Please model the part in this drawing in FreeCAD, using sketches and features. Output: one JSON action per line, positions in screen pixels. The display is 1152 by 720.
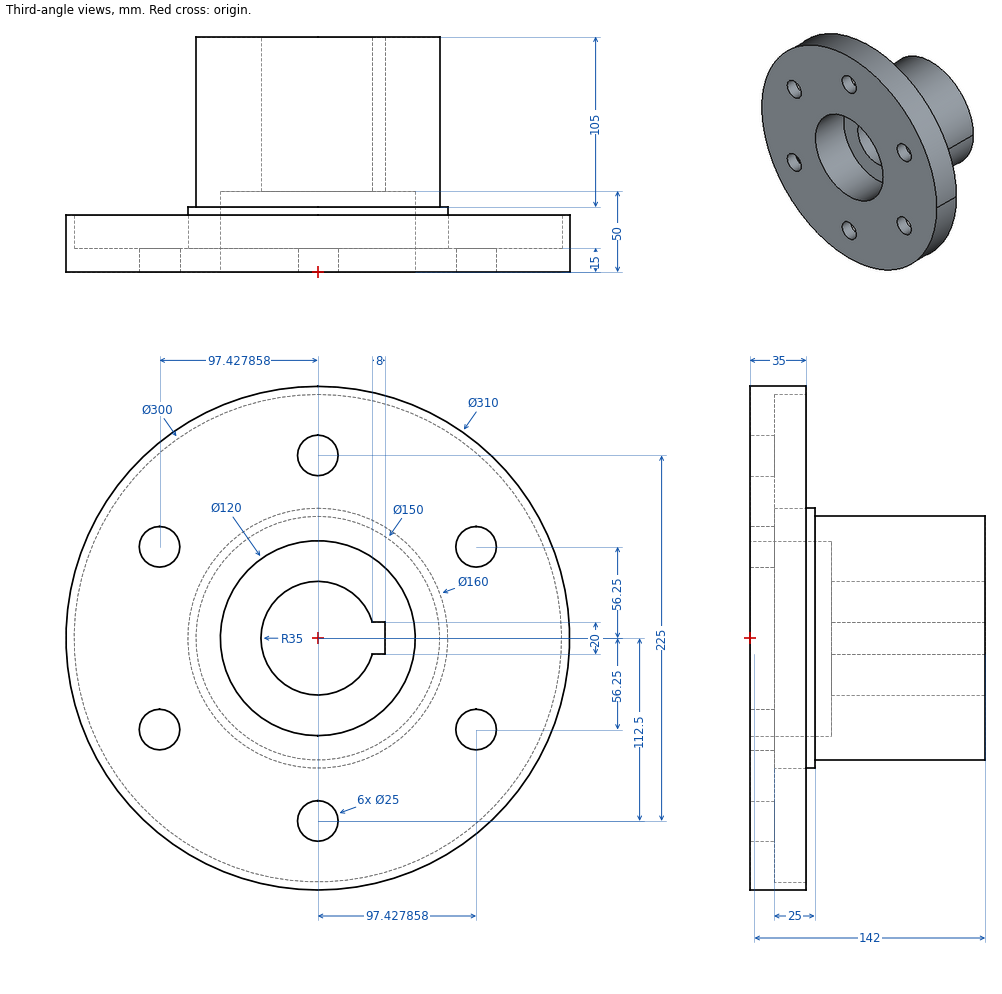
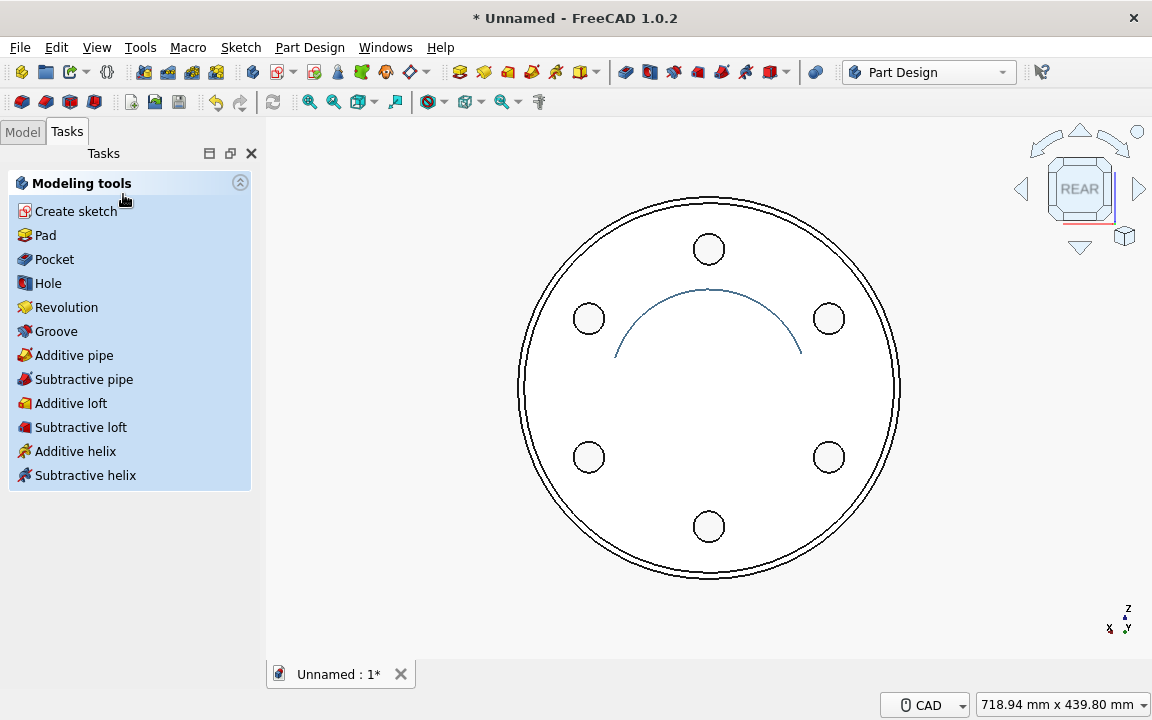
{"action": "left_click", "coordinate": [460, 72]}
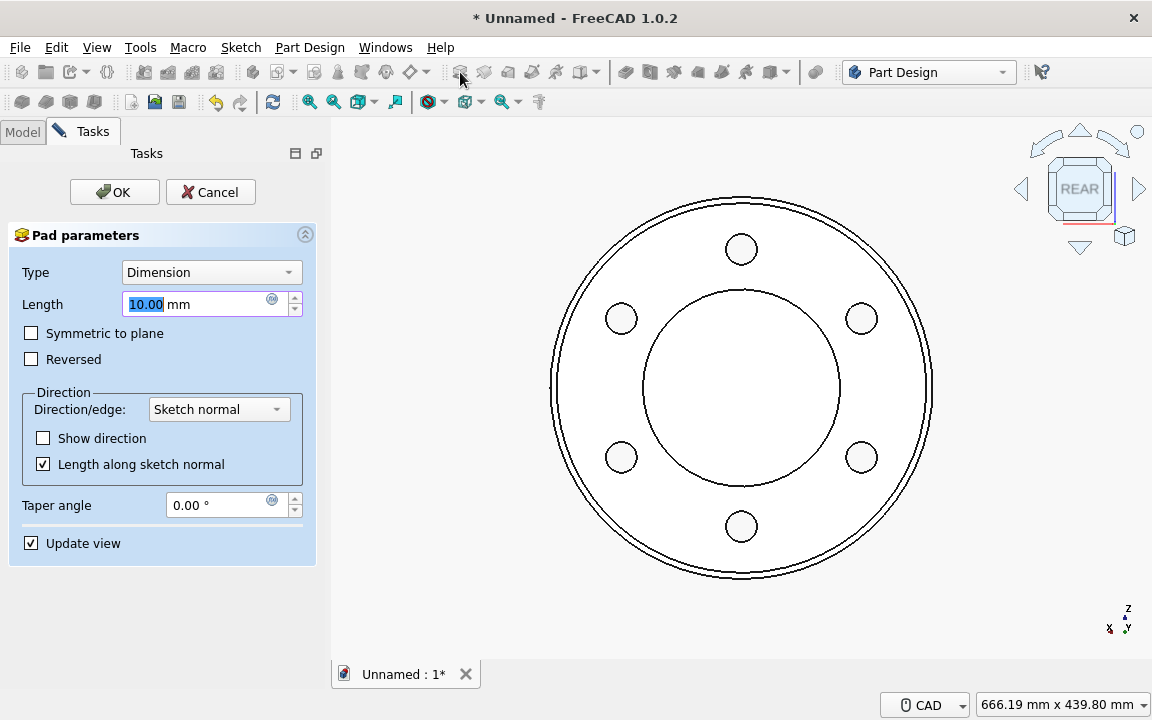
{"action": "type", "text": "25"}
{"action": "key", "text": "Tab"}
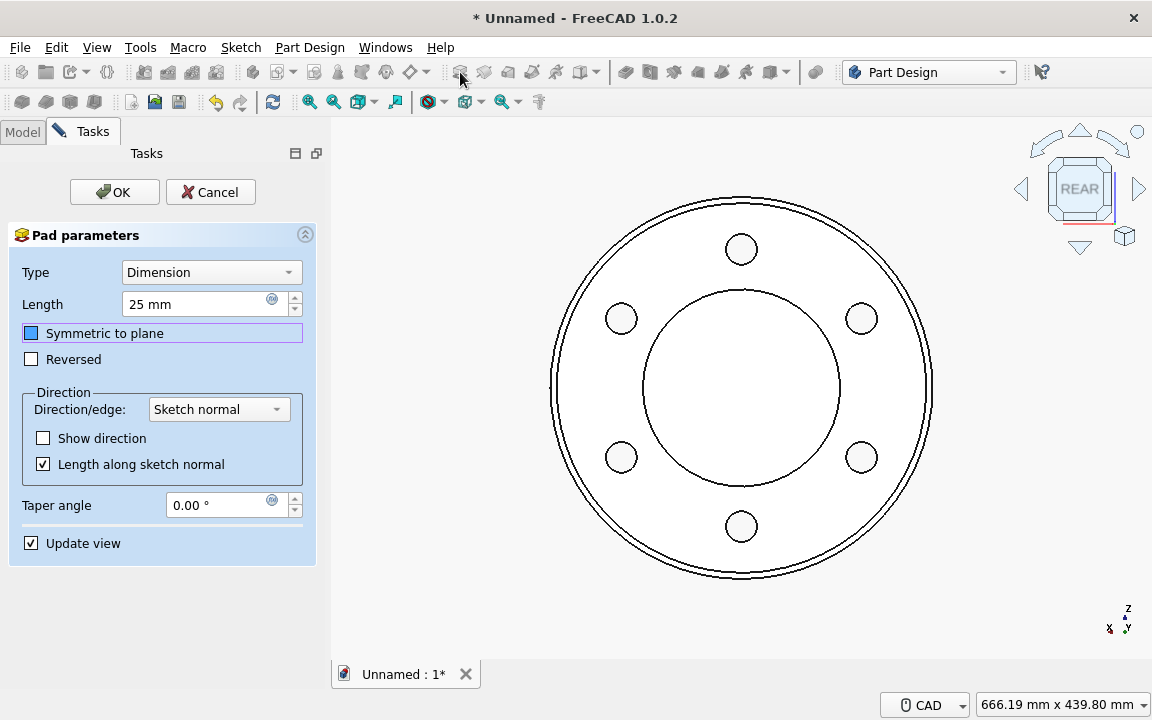
{"action": "left_click", "coordinate": [115, 192]}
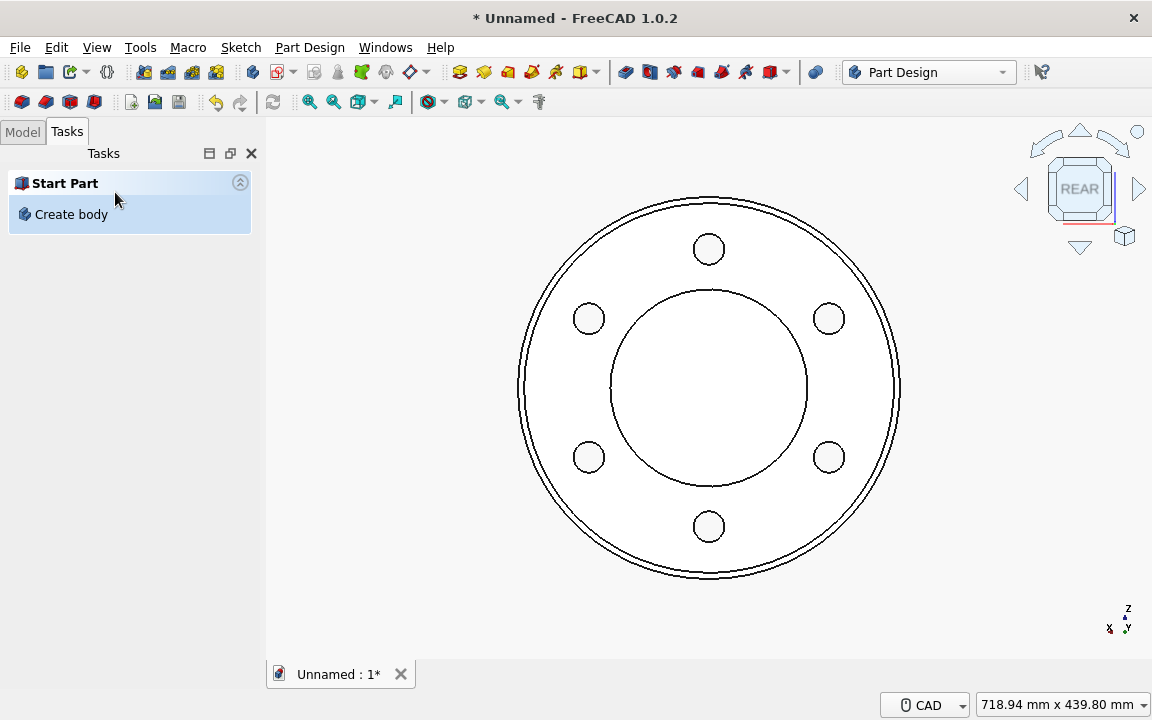
{"action": "left_click", "coordinate": [709, 387]}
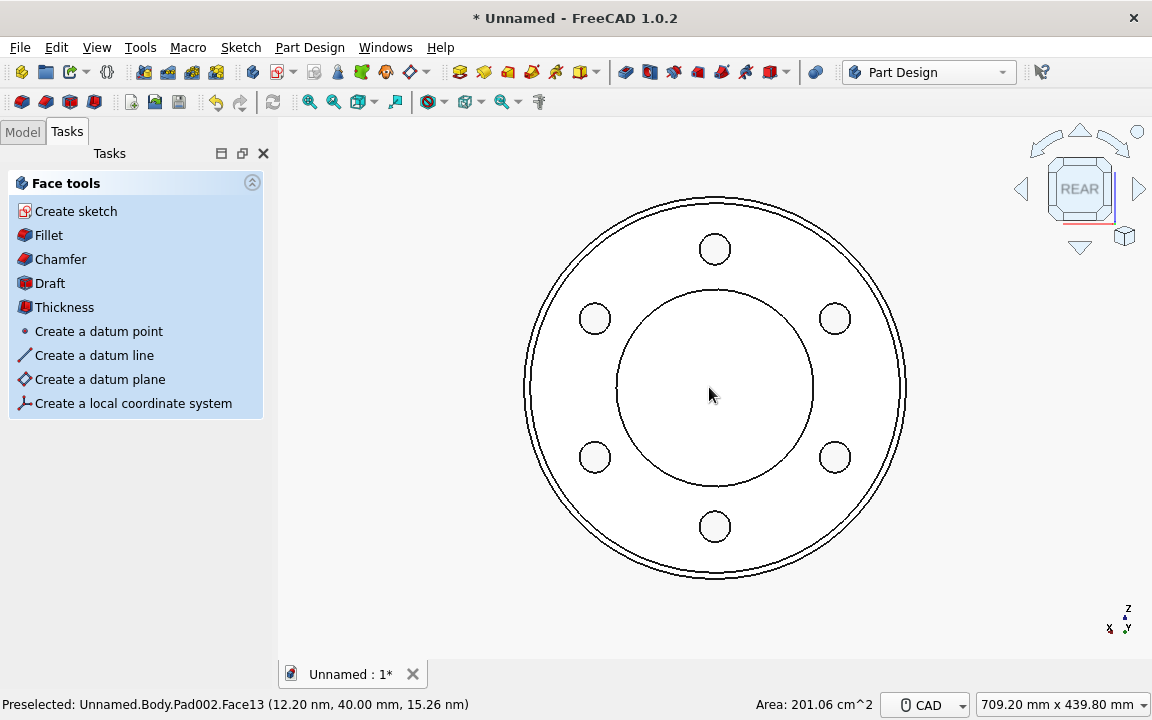
{"action": "left_click", "coordinate": [278, 72]}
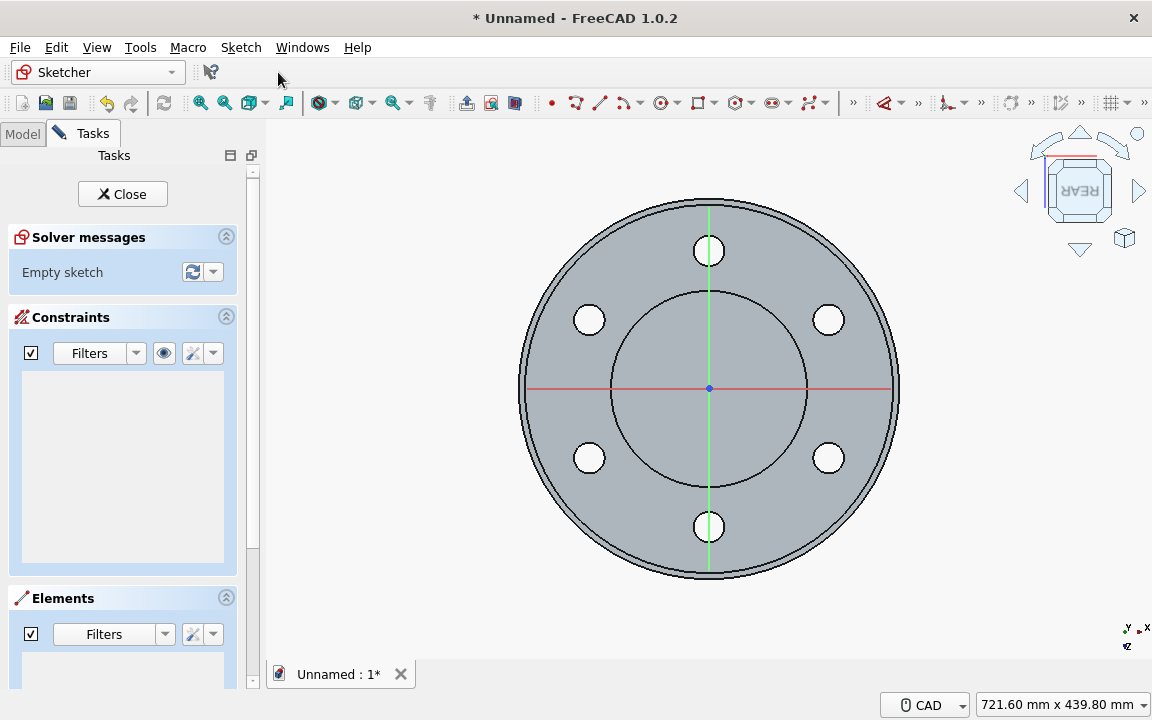
{"action": "scroll", "coordinate": [792, 389], "scroll_direction": "up", "scroll_amount": 3}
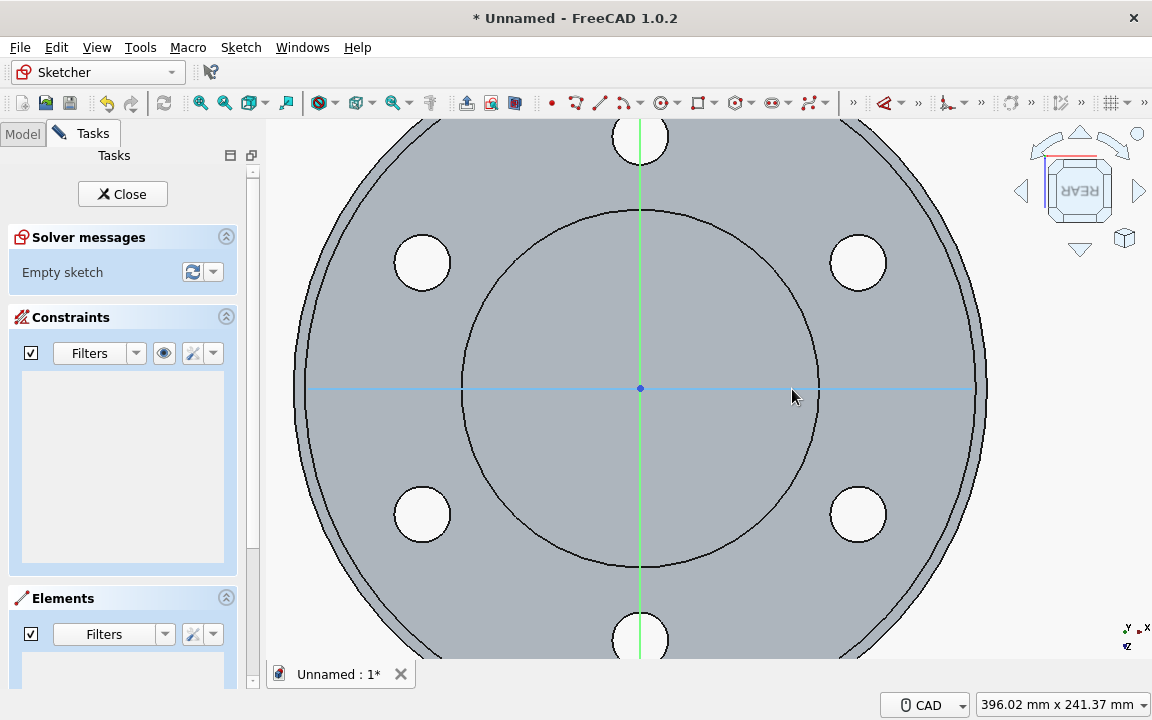
{"action": "left_click", "coordinate": [662, 104]}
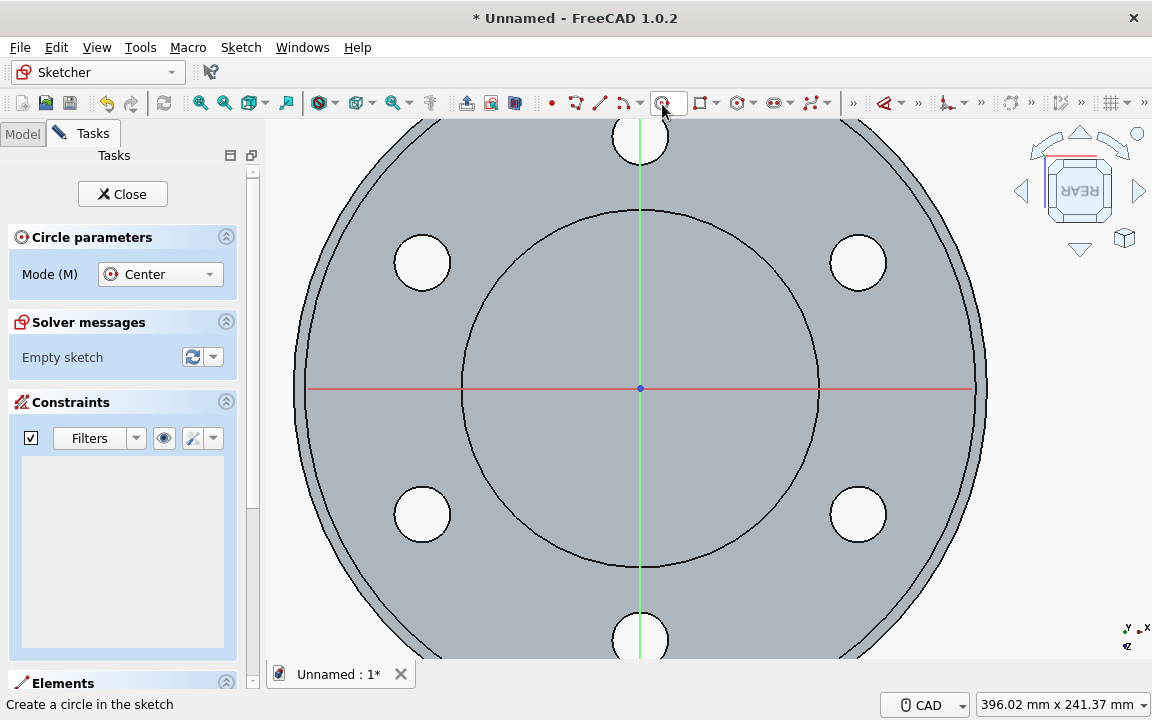
{"action": "left_click", "coordinate": [640, 389]}
{"action": "mouse_move", "coordinate": [759, 270]}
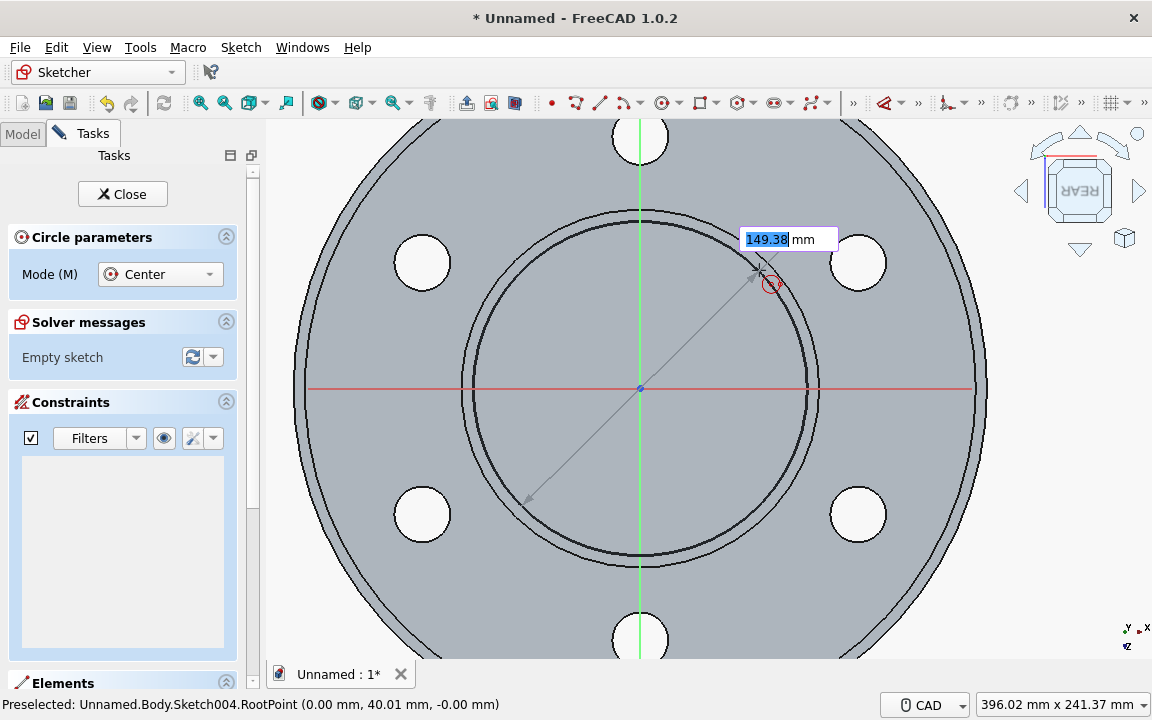
{"action": "type", "text": "150"}
{"action": "key", "text": "Return"}
{"action": "key", "text": "Escape"}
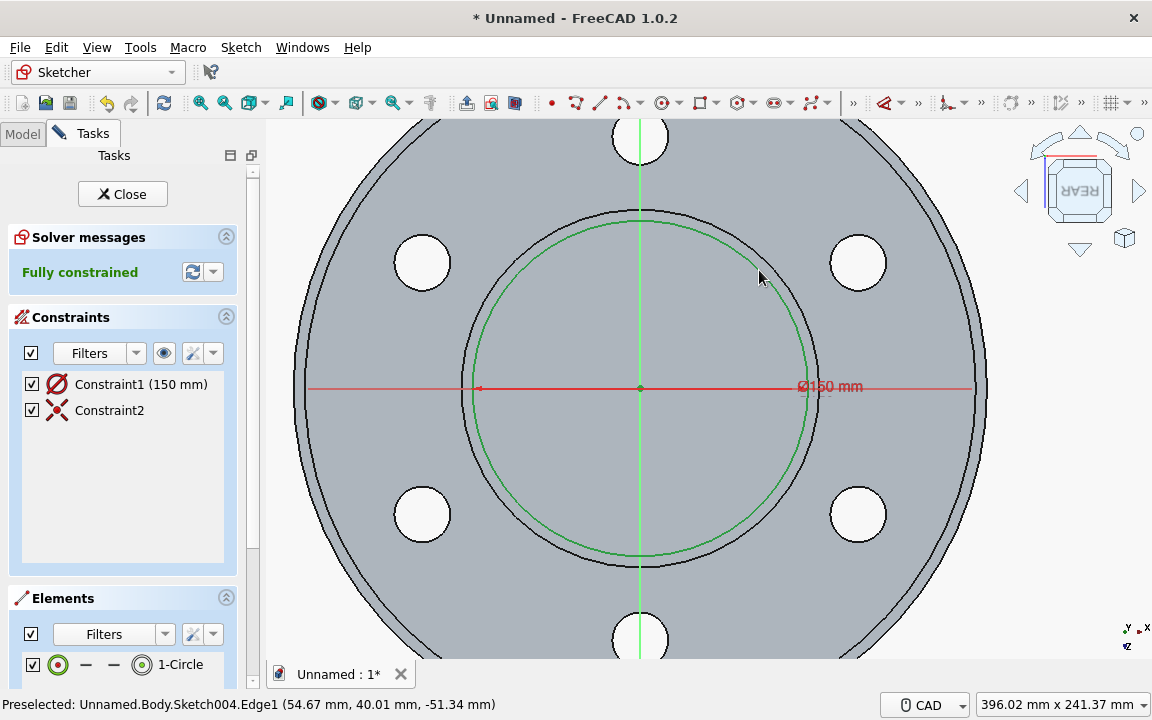
{"action": "left_click", "coordinate": [123, 194]}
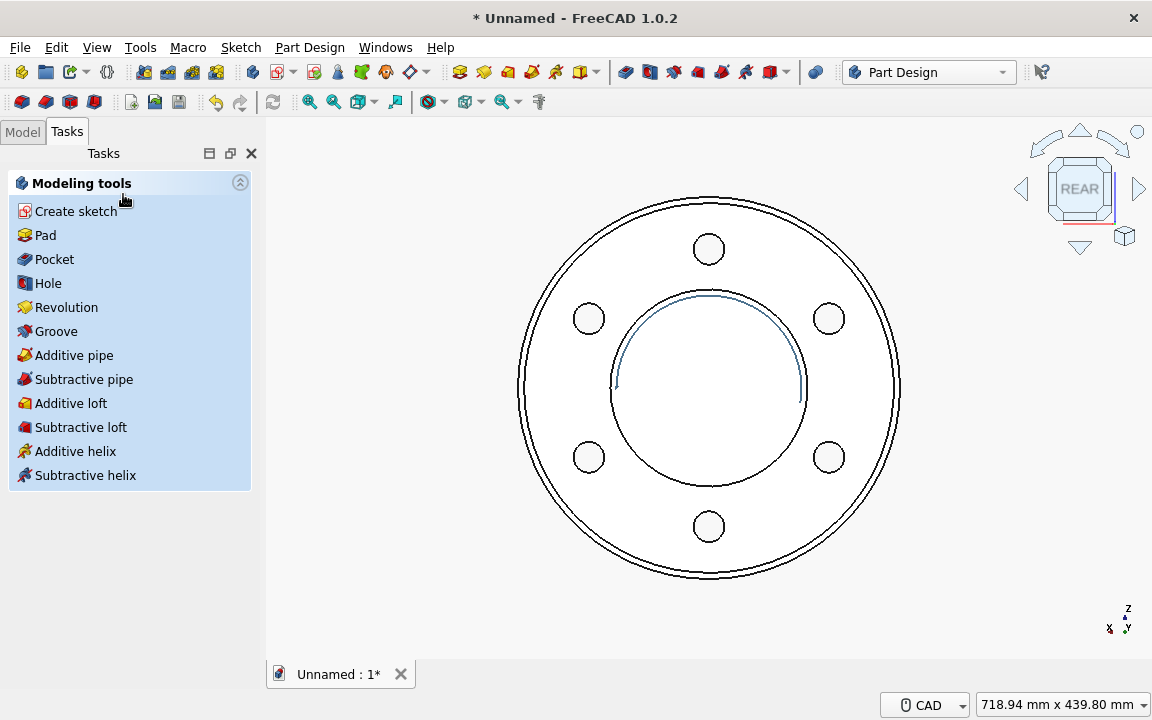
{"action": "left_click", "coordinate": [460, 72]}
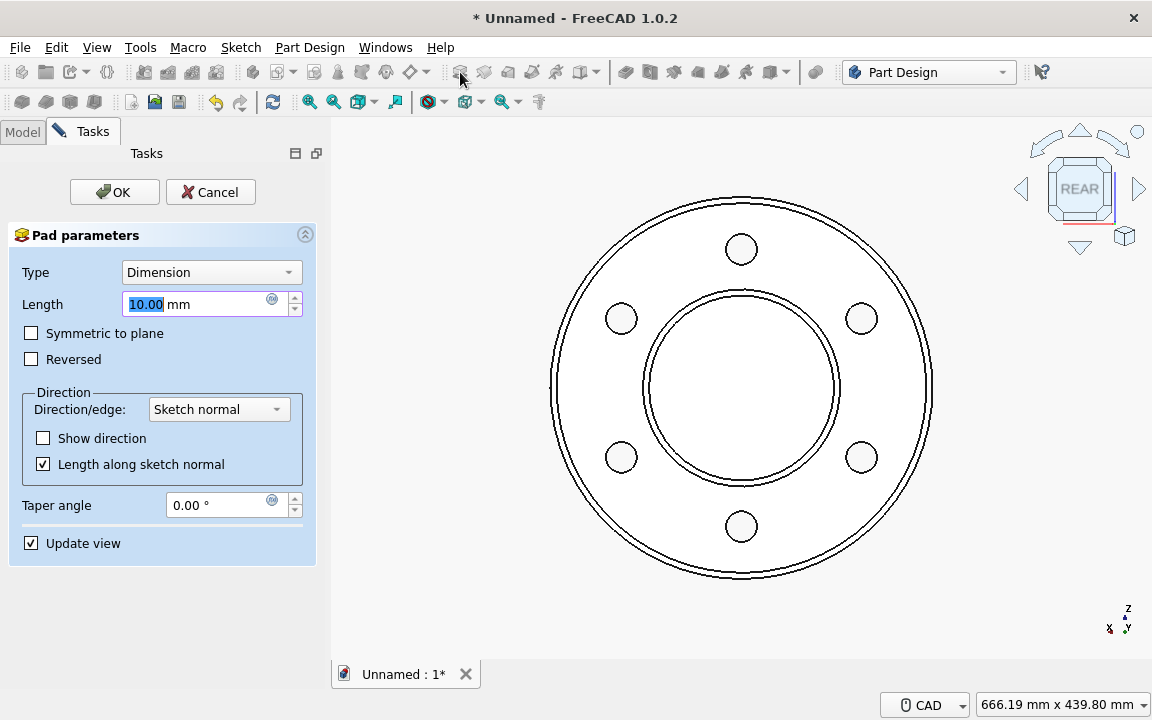
{"action": "type", "text": "105"}
{"action": "key", "text": "Tab"}